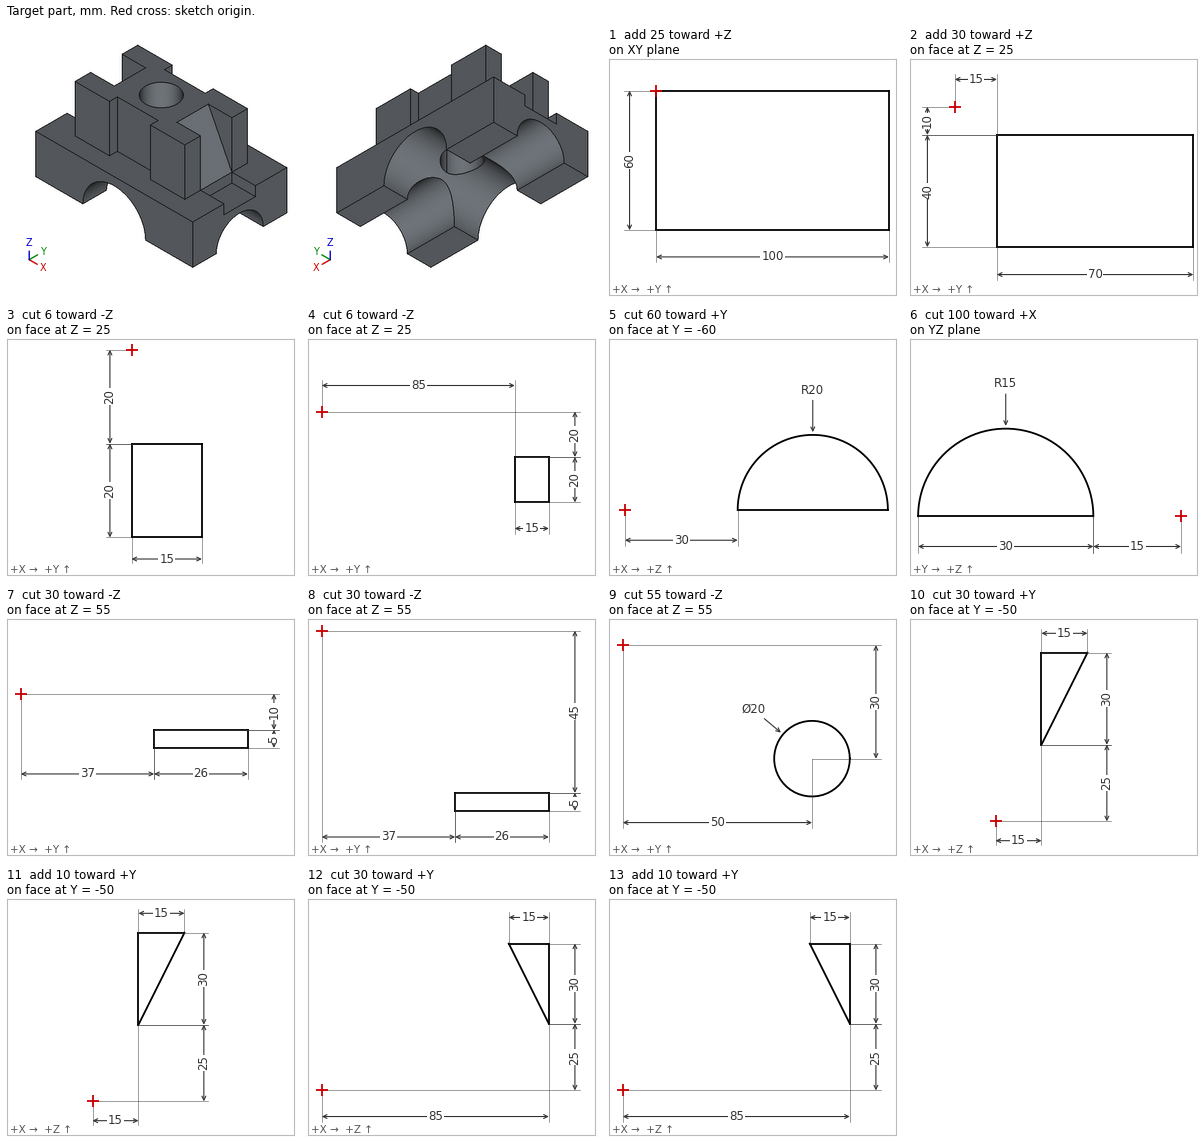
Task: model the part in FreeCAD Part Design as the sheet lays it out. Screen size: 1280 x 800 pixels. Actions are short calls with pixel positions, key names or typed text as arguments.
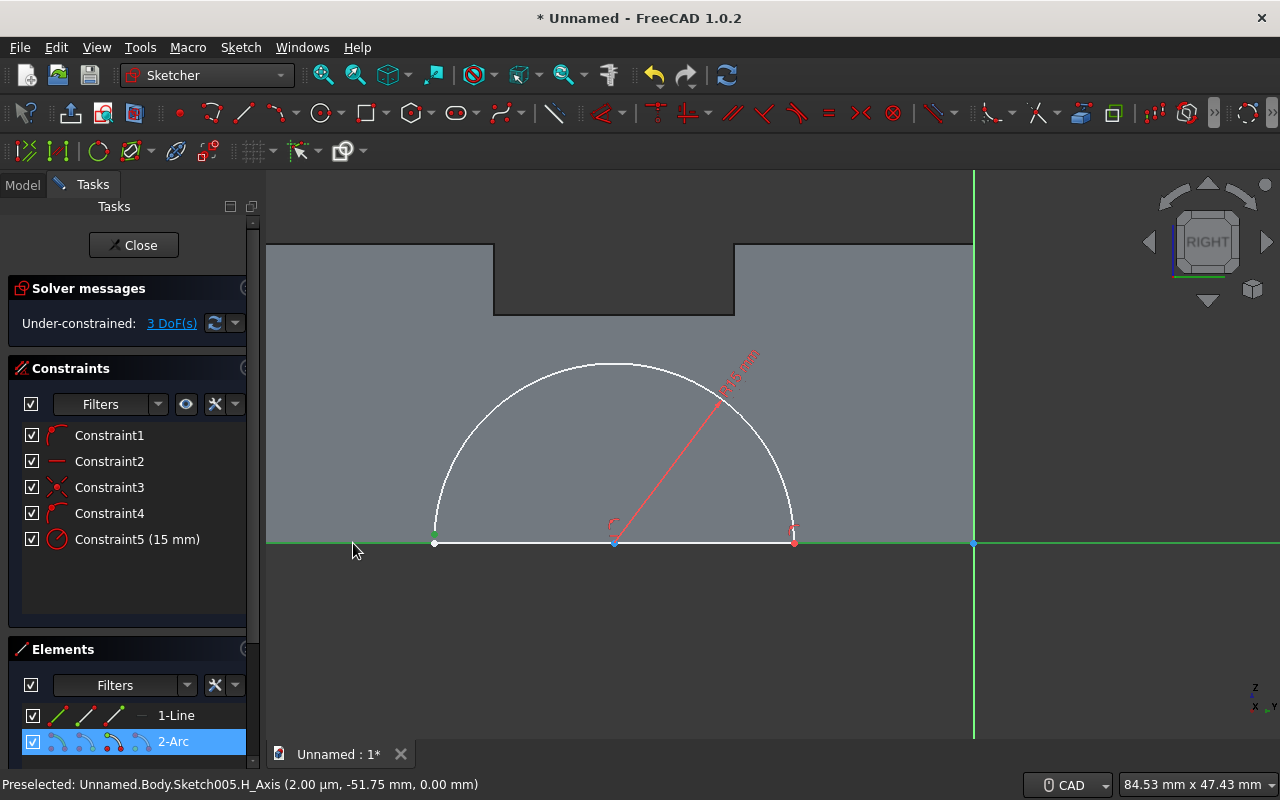
click(656, 114)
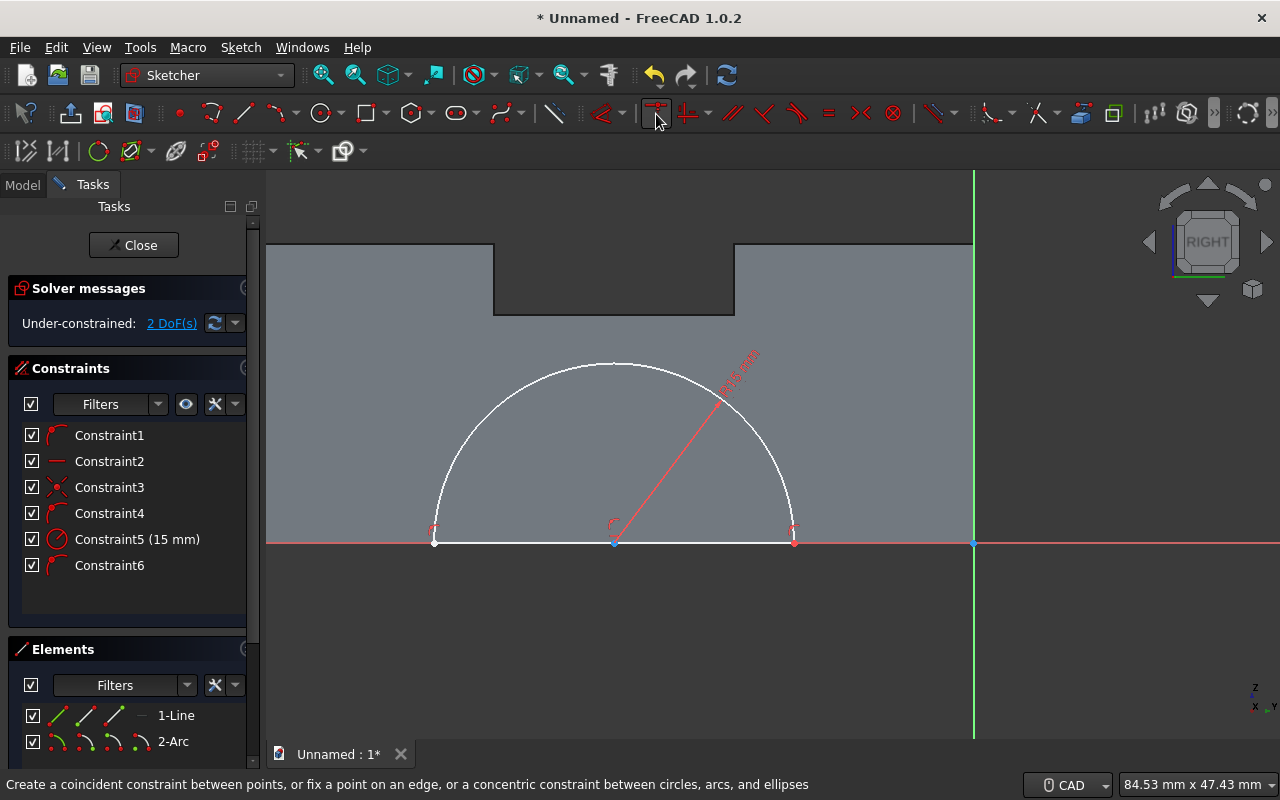
key(d)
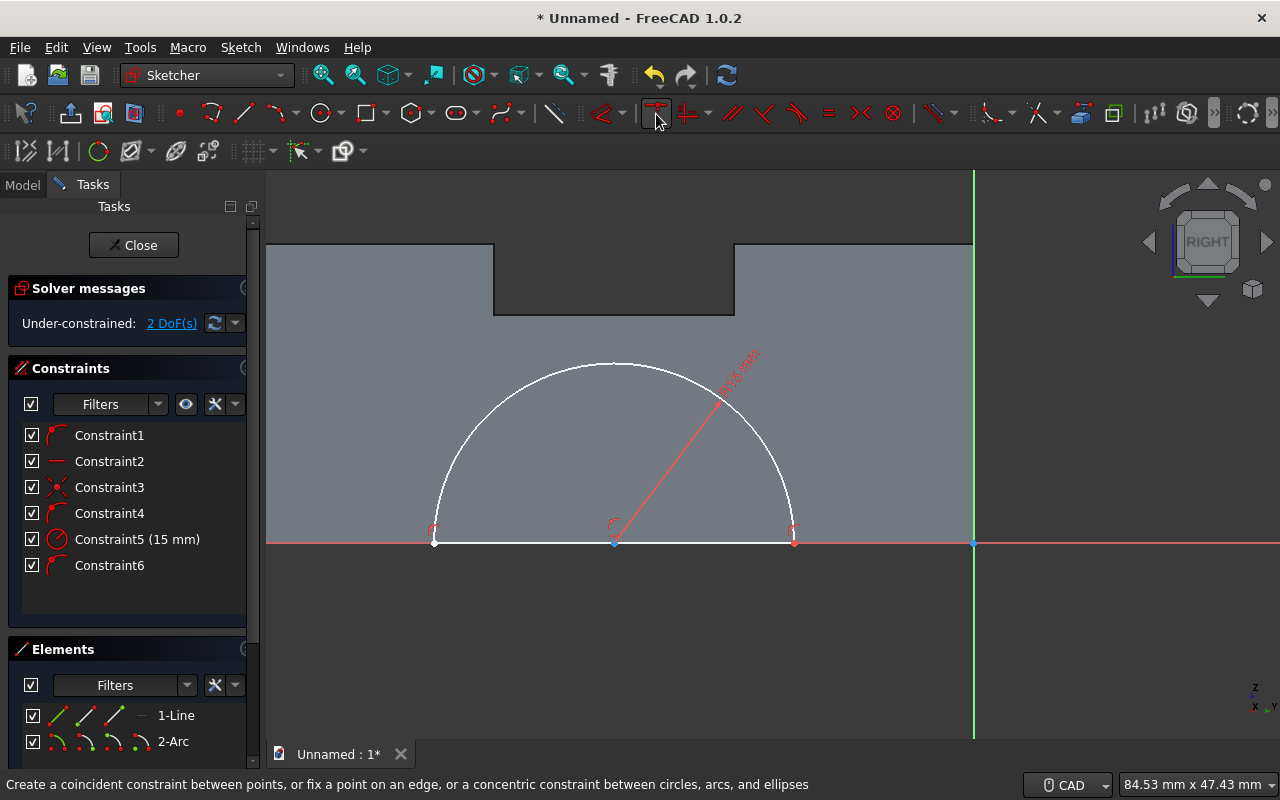
click(686, 543)
click(614, 577)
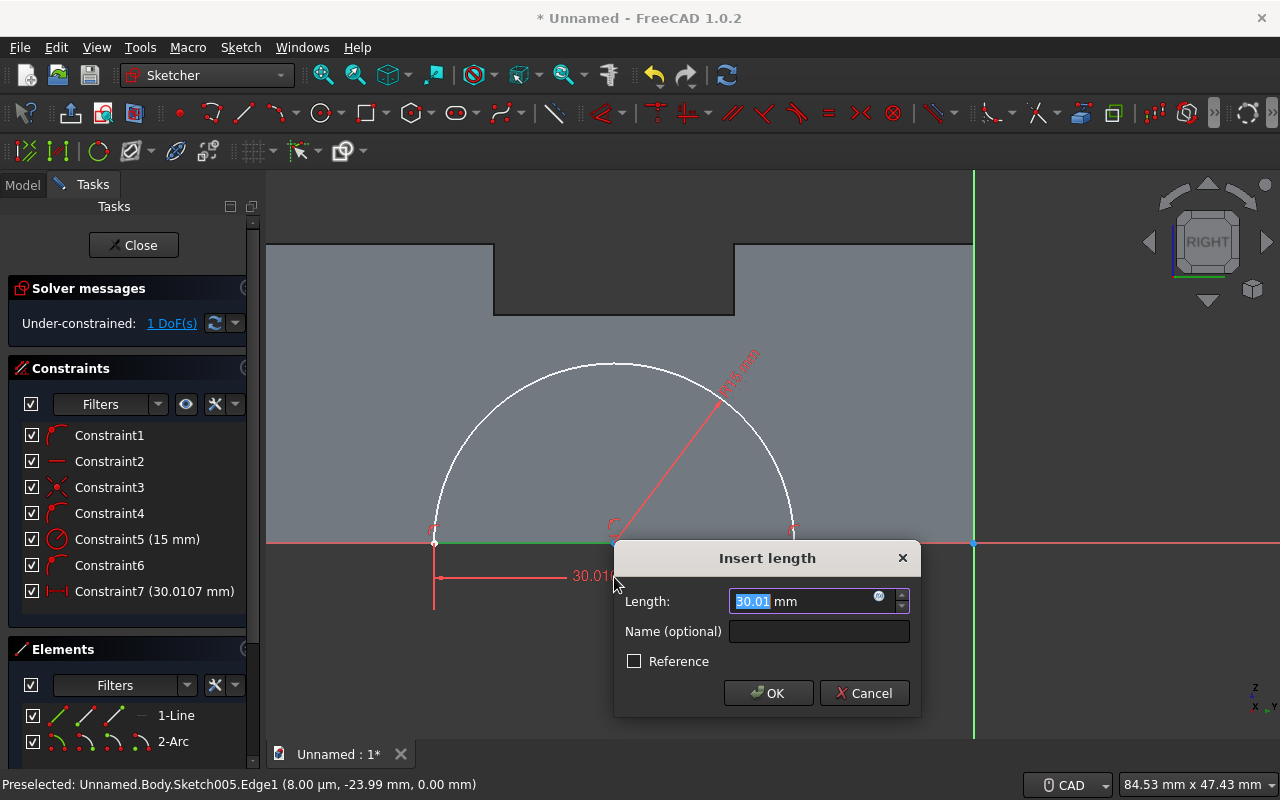
text(30)
key(Return)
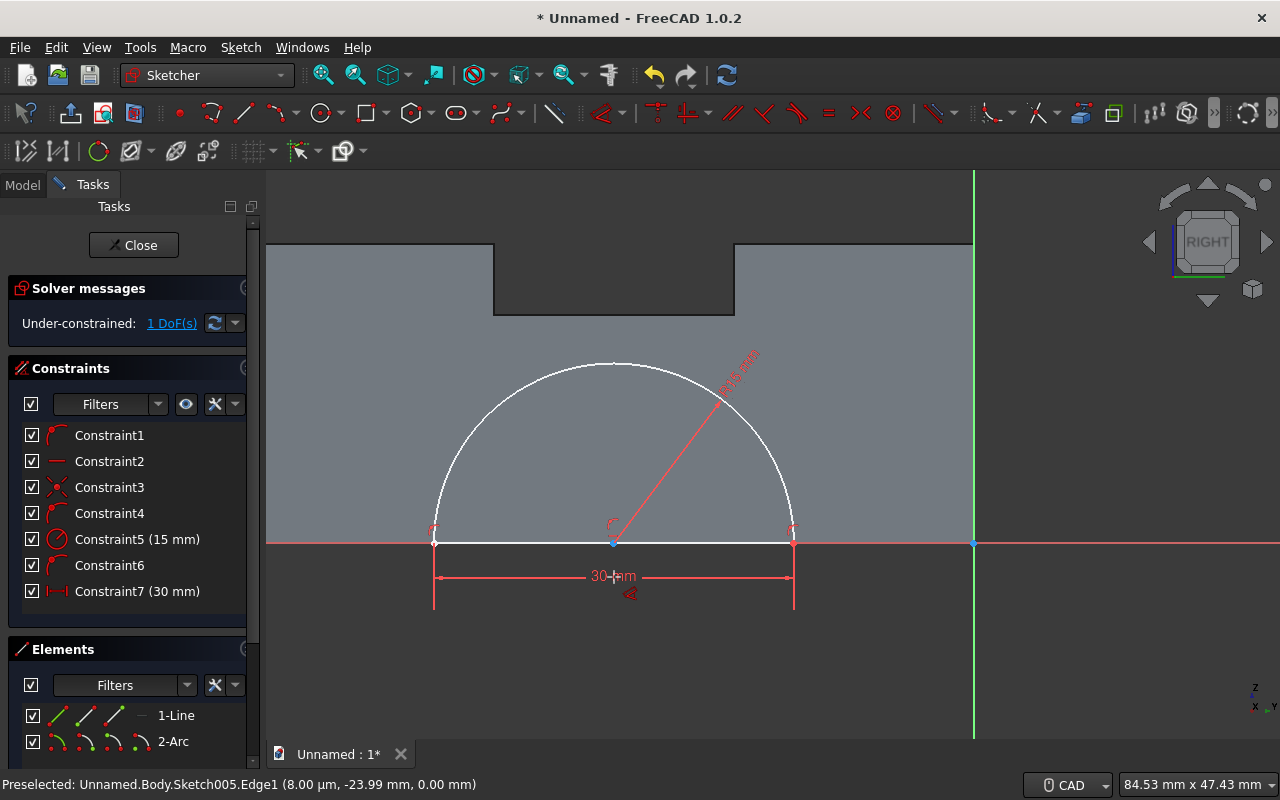
click(794, 543)
click(884, 577)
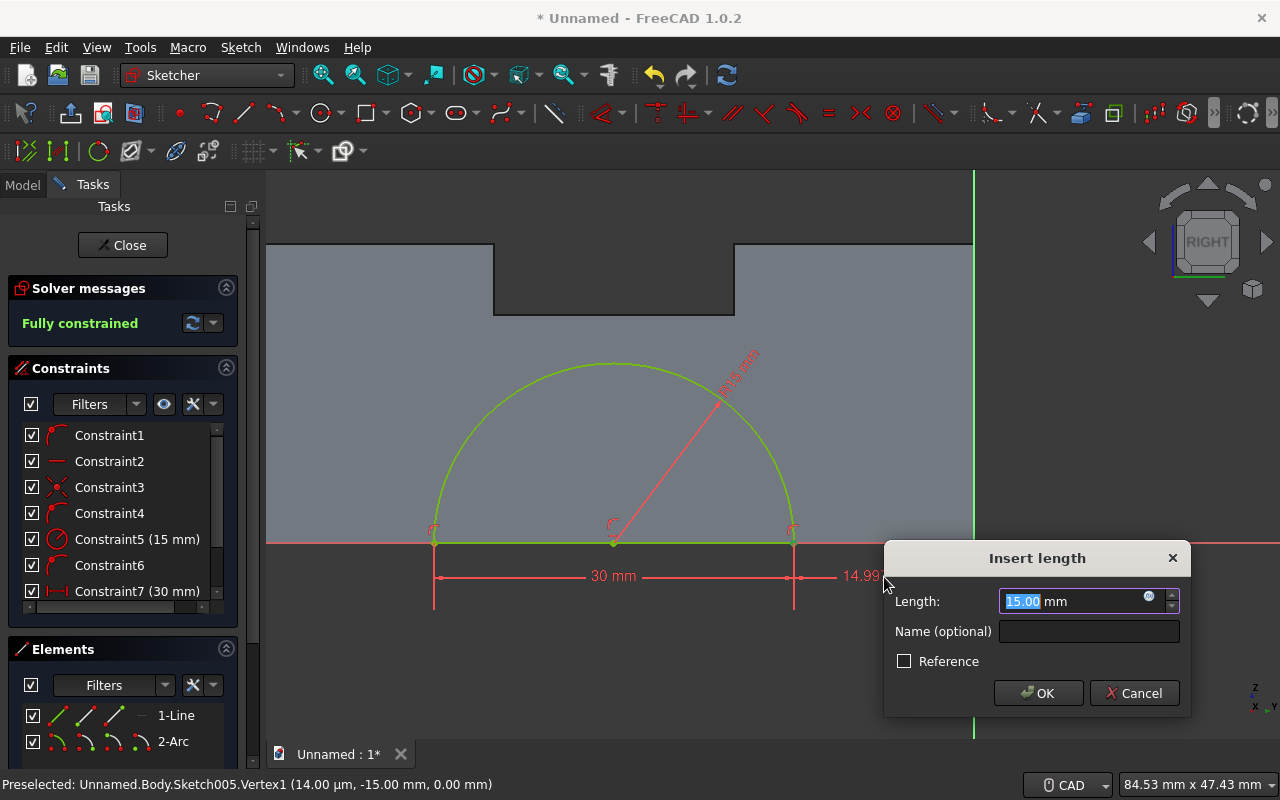
text(15)
key(Return)
key(Escape)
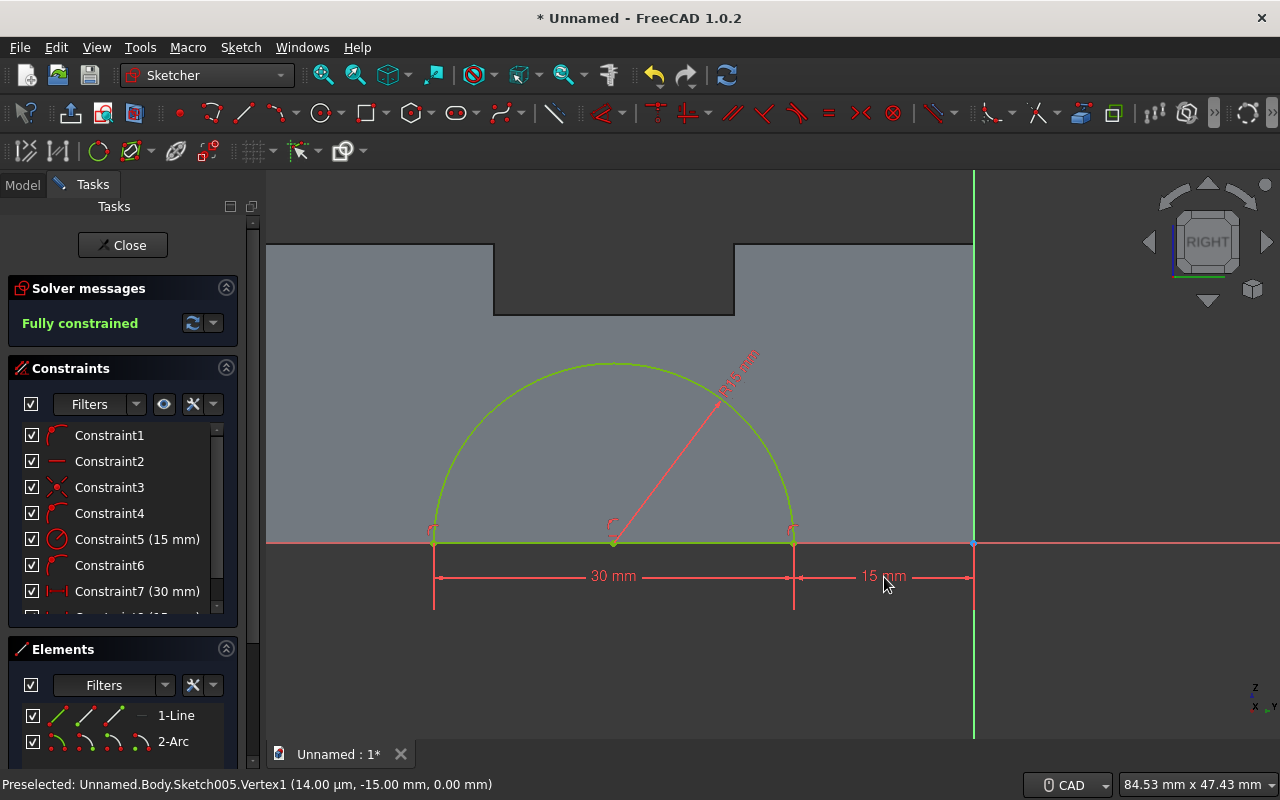
click(123, 245)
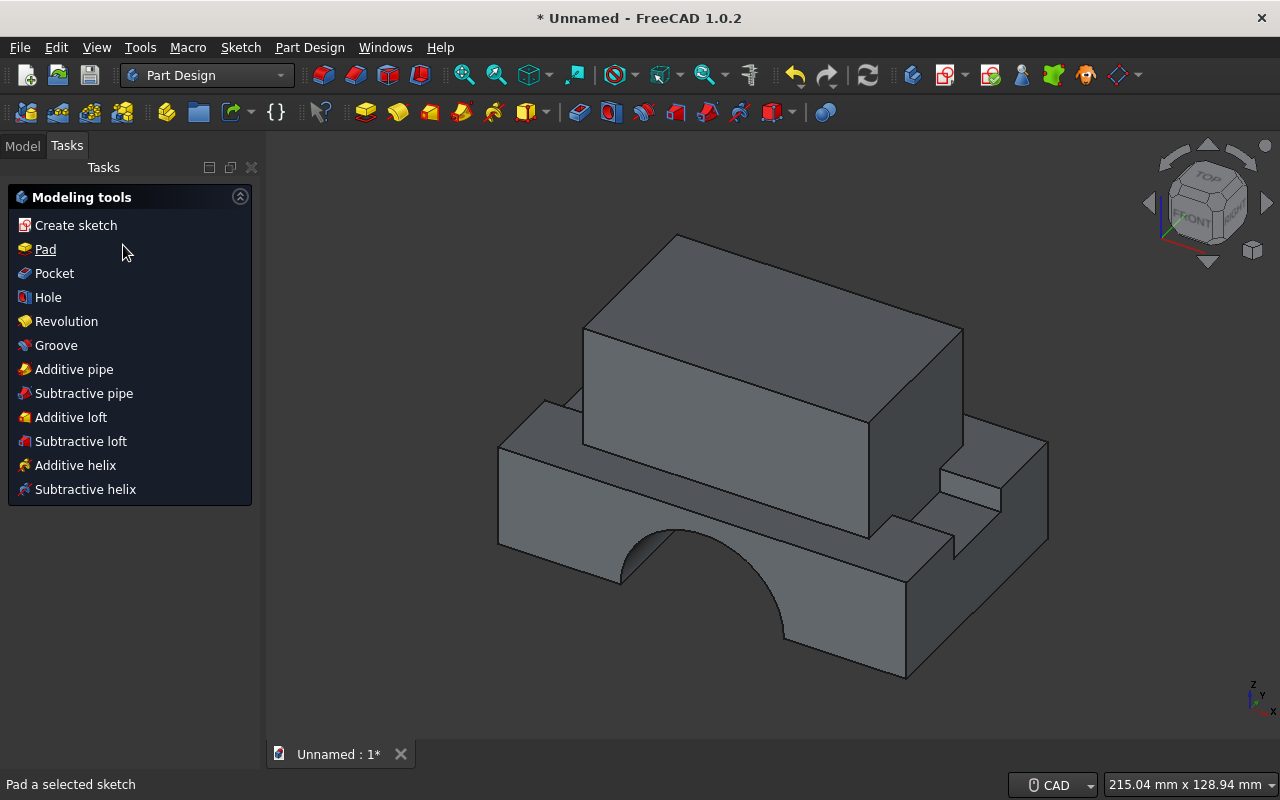
click(580, 112)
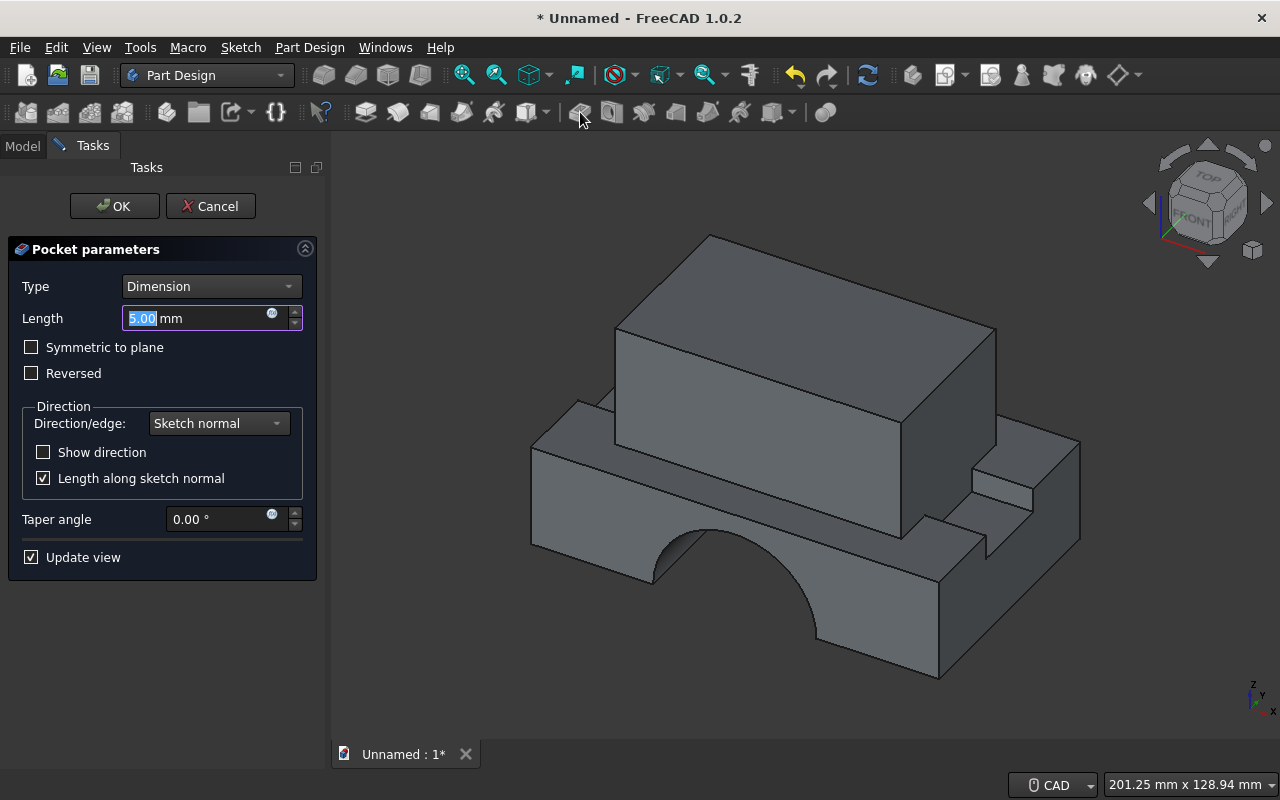
text(100)
key(Tab)